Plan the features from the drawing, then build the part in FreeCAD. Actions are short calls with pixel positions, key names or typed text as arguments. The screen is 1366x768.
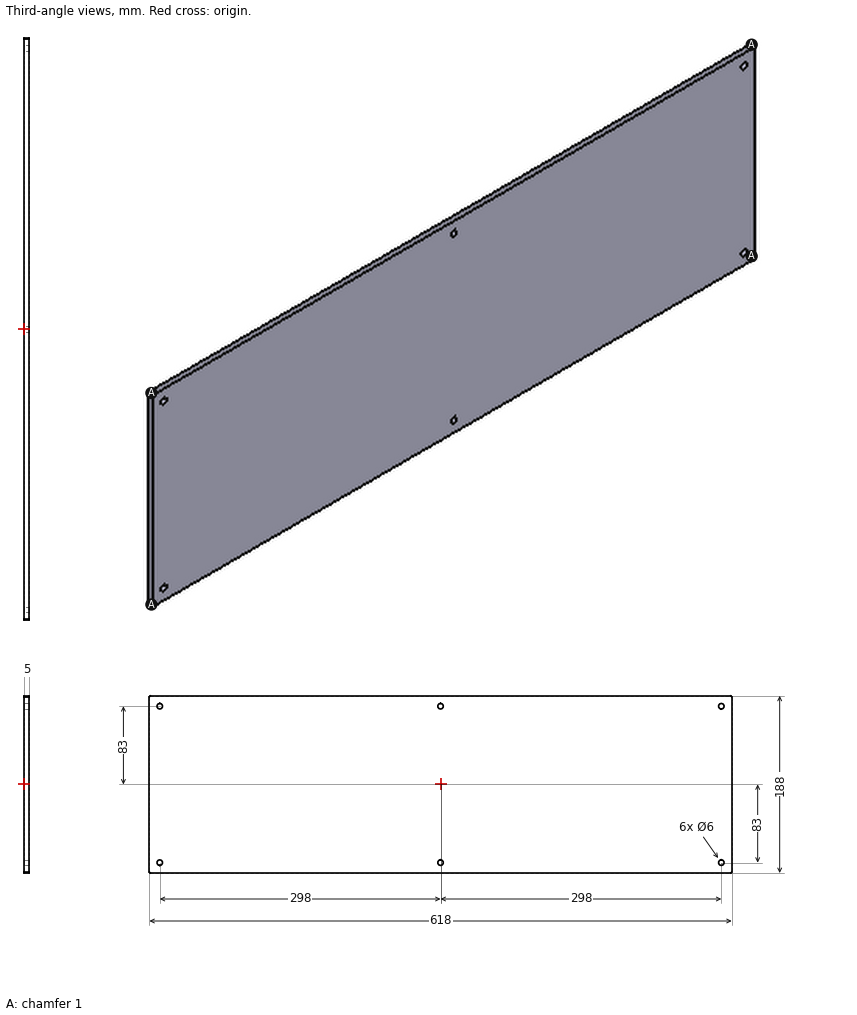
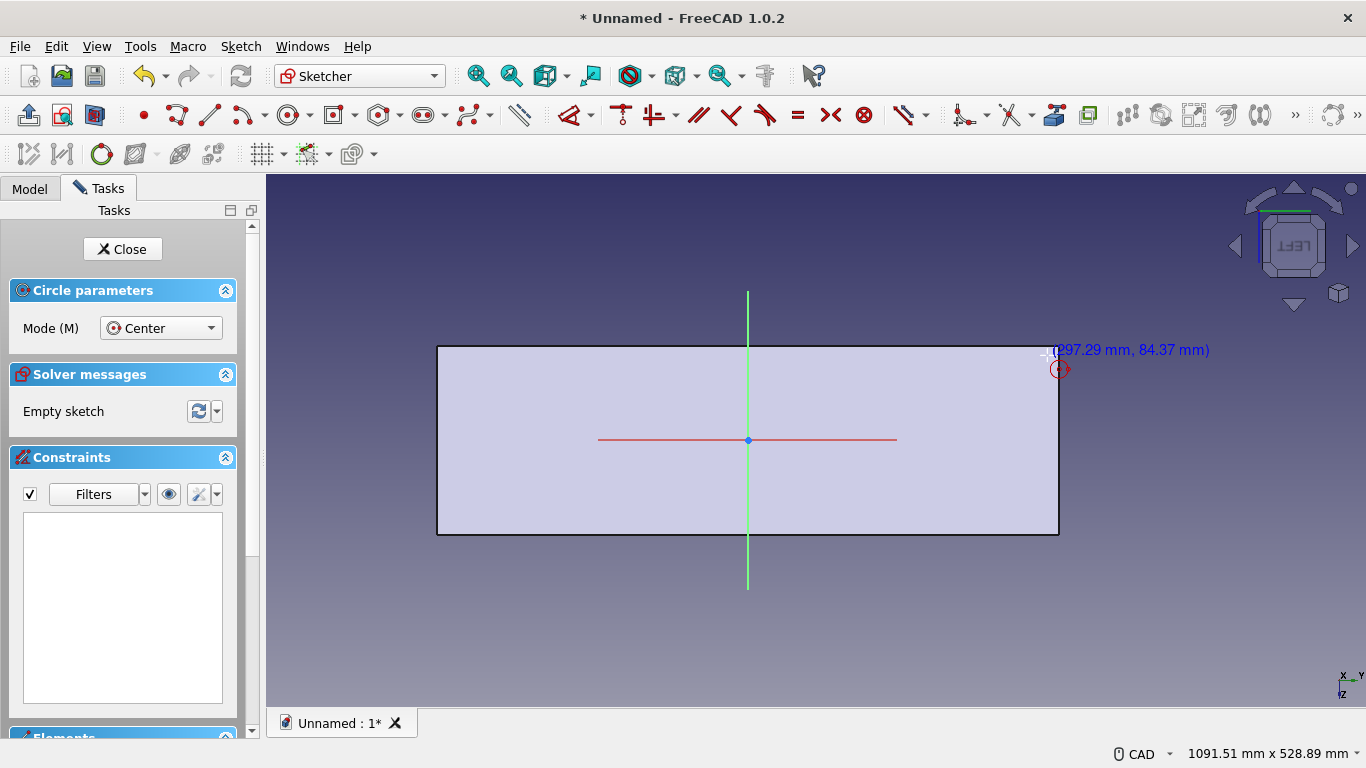
click(1048, 357)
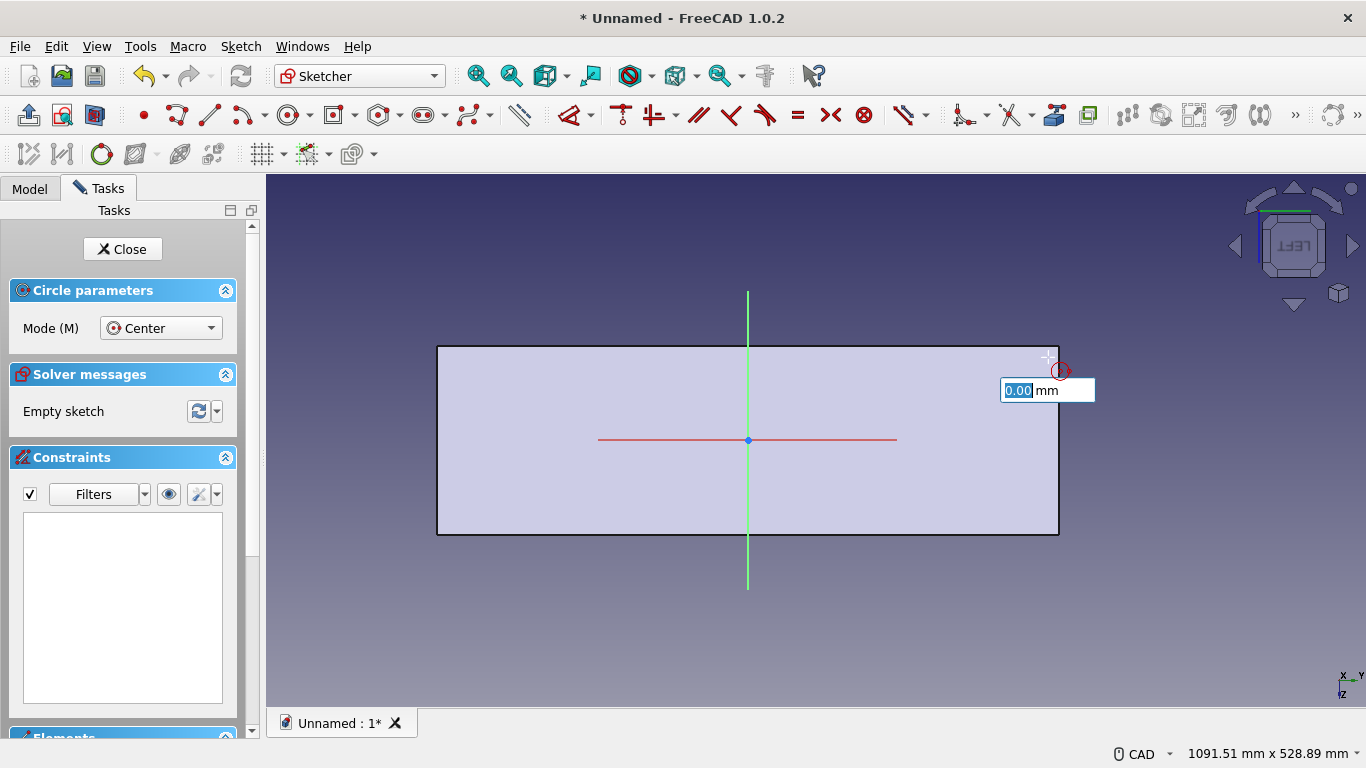
scroll(1050, 355, up, 9)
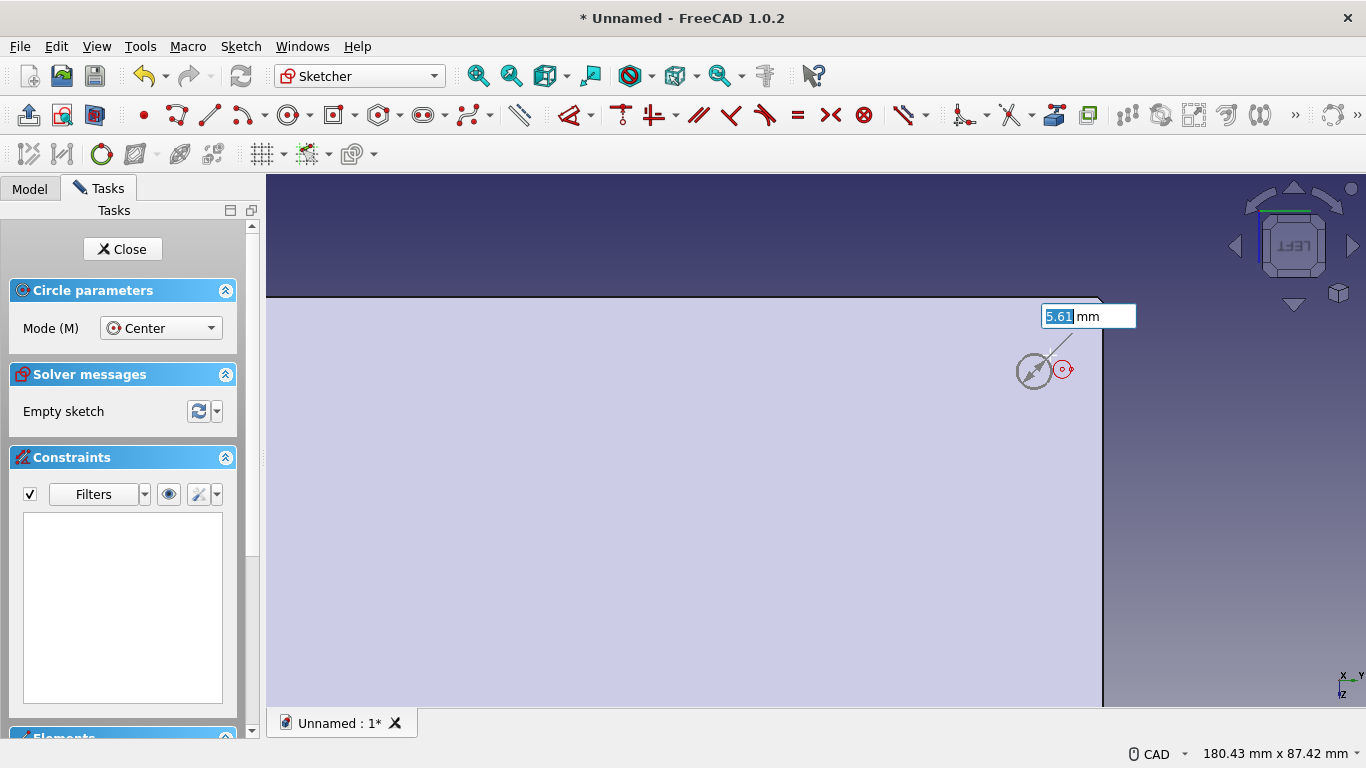
click(1049, 351)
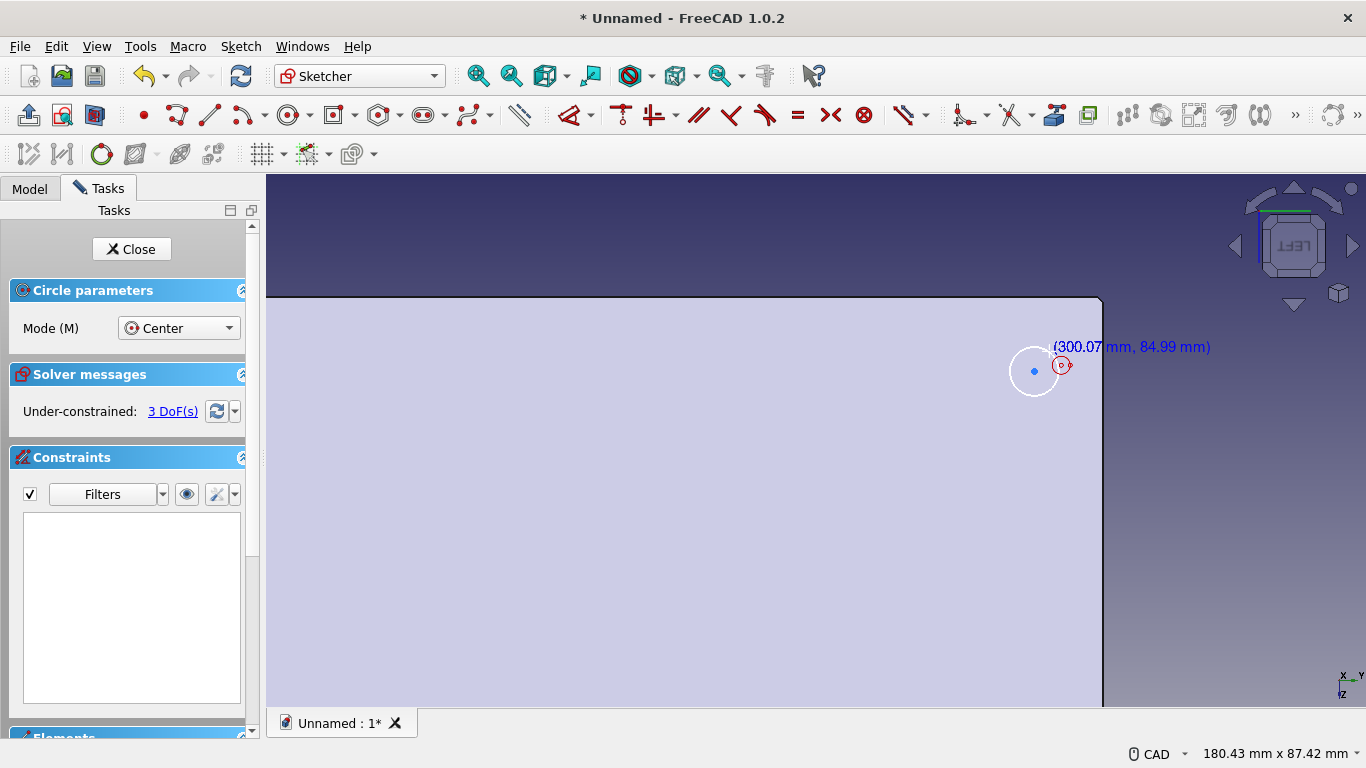
scroll(1050, 355, down, 9)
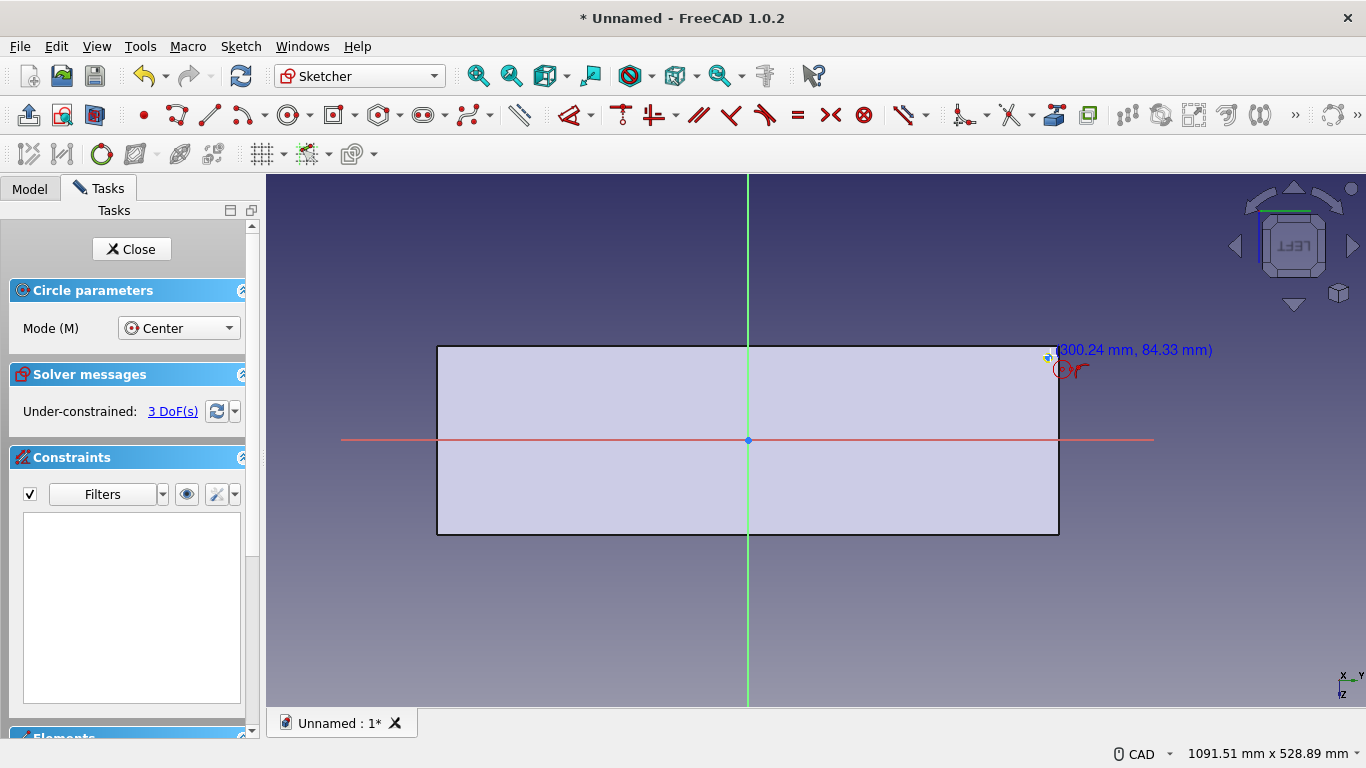
scroll(448, 357, up, 11)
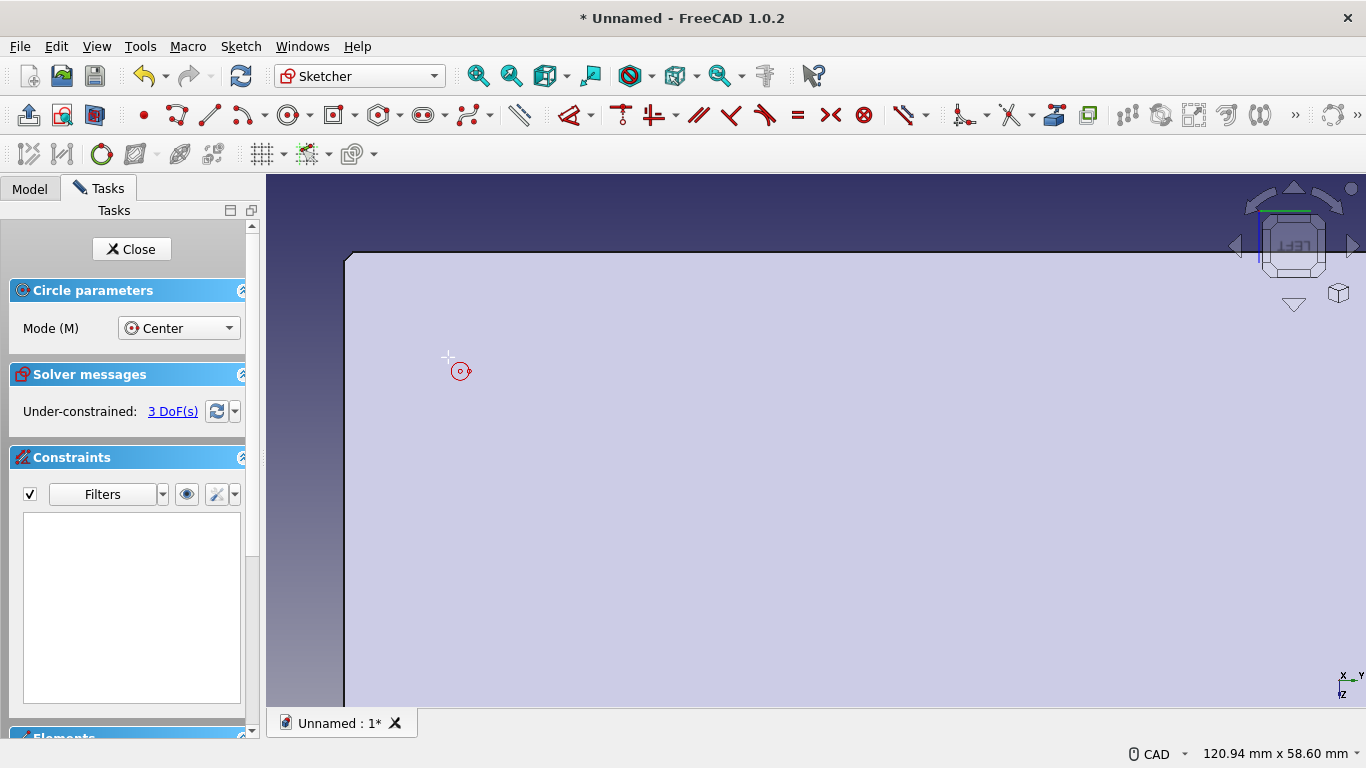
scroll(448, 357, down, 11)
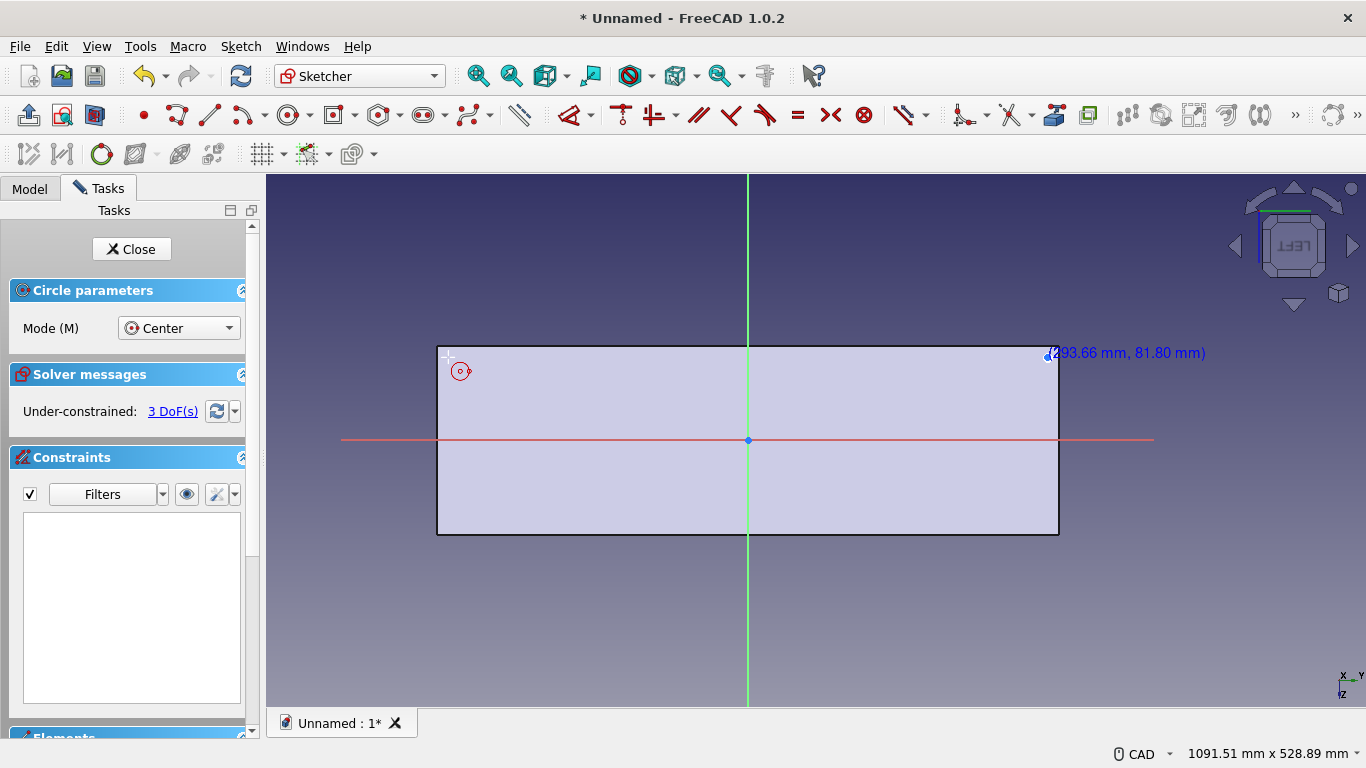
click(448, 357)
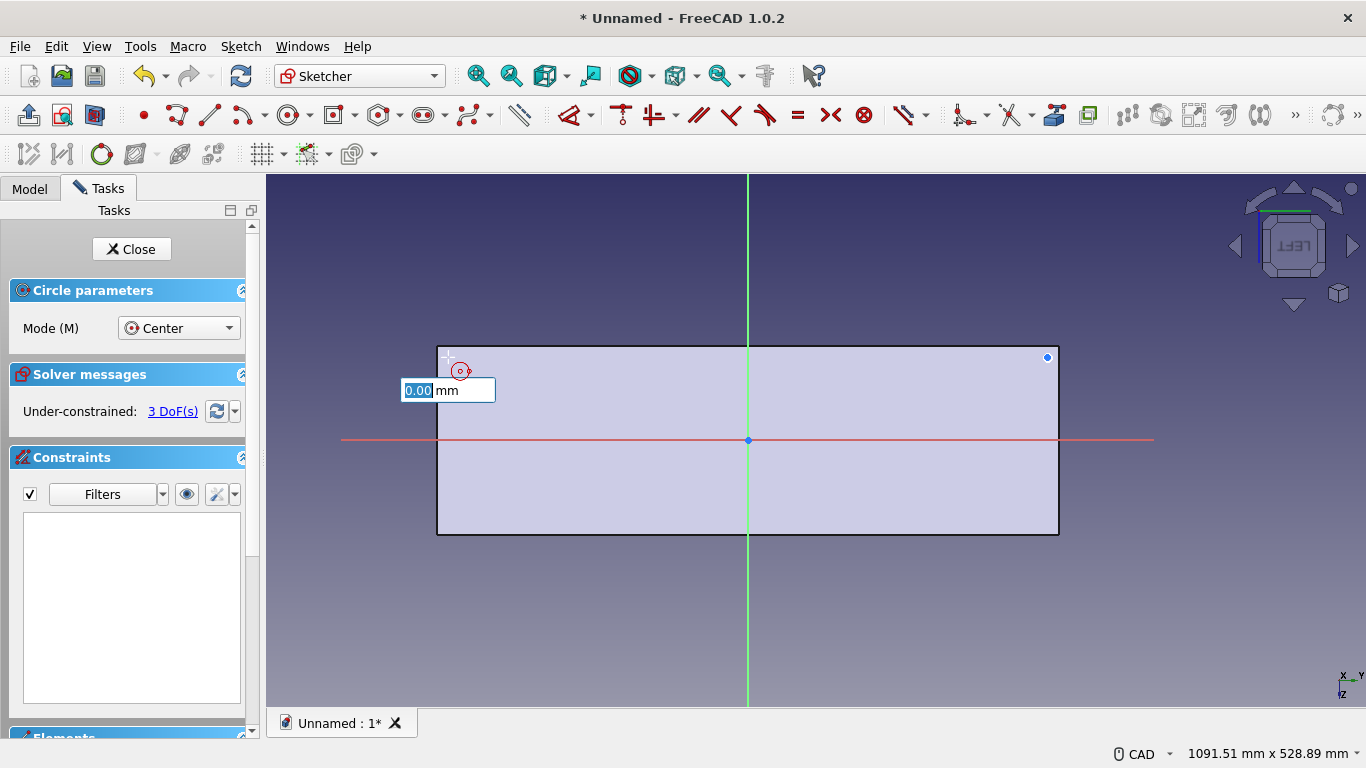
scroll(450, 355, up, 9)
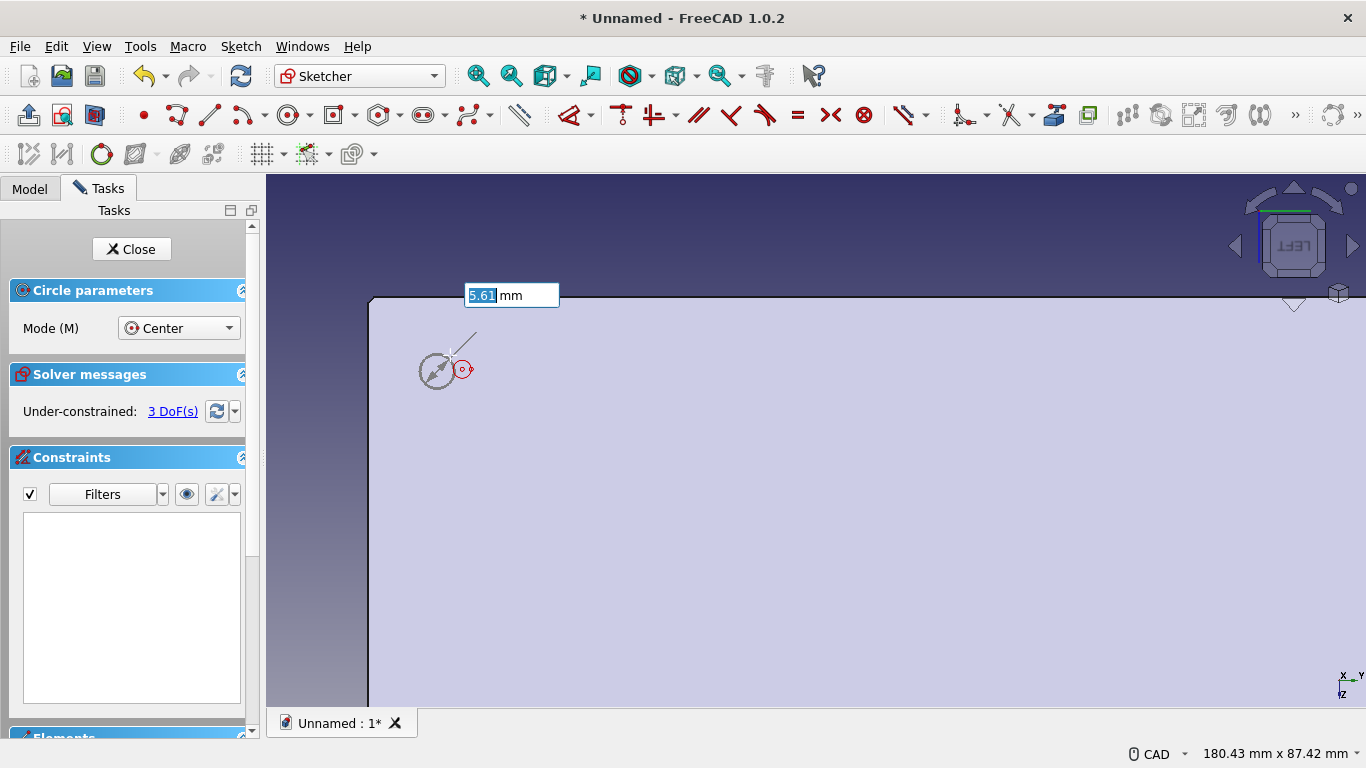
click(448, 351)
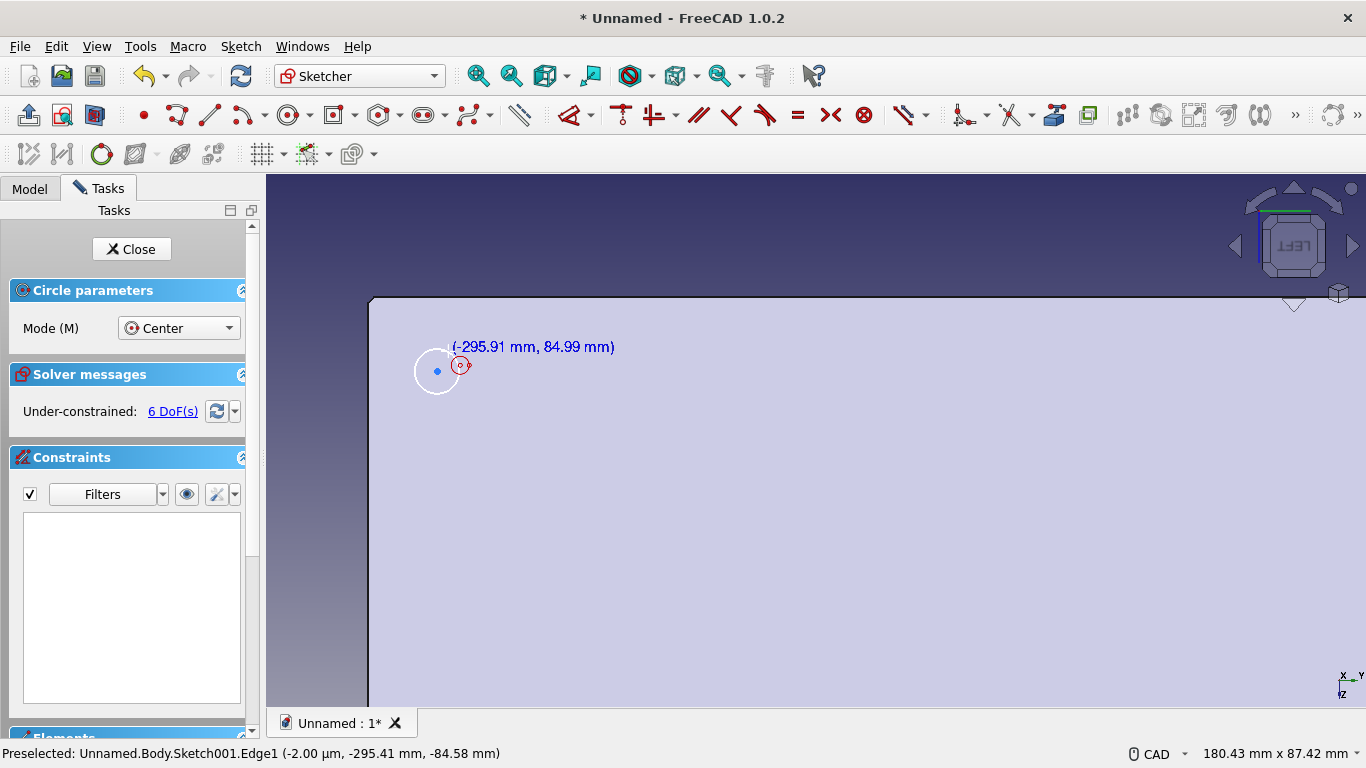
scroll(450, 355, down, 9)